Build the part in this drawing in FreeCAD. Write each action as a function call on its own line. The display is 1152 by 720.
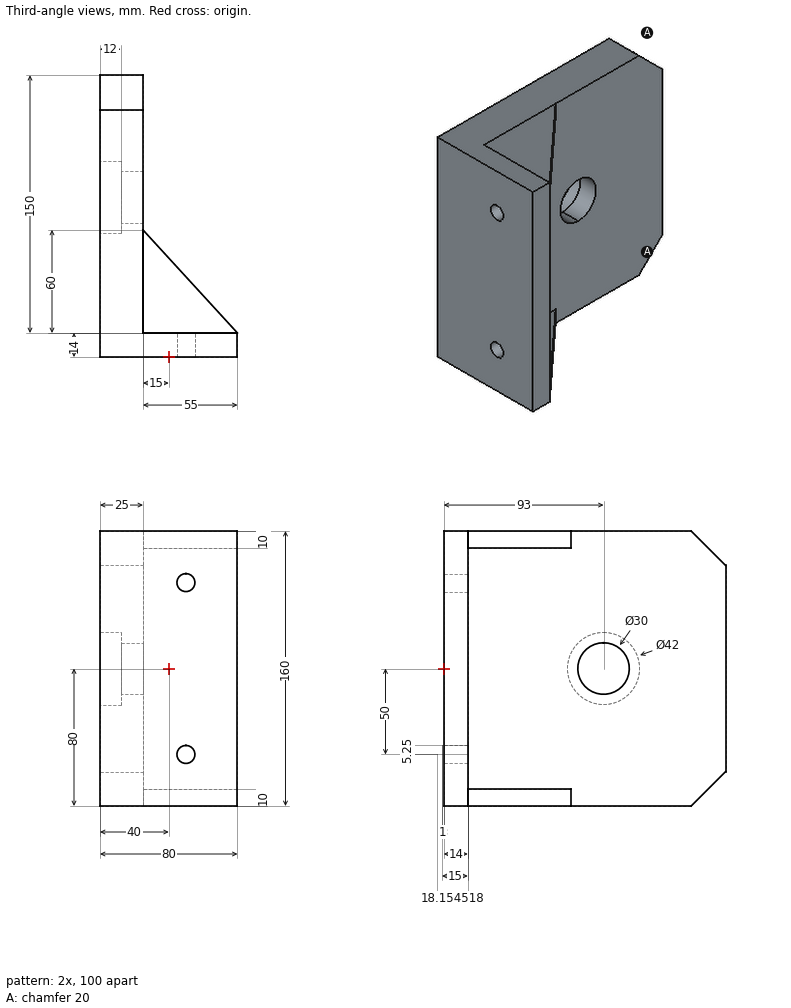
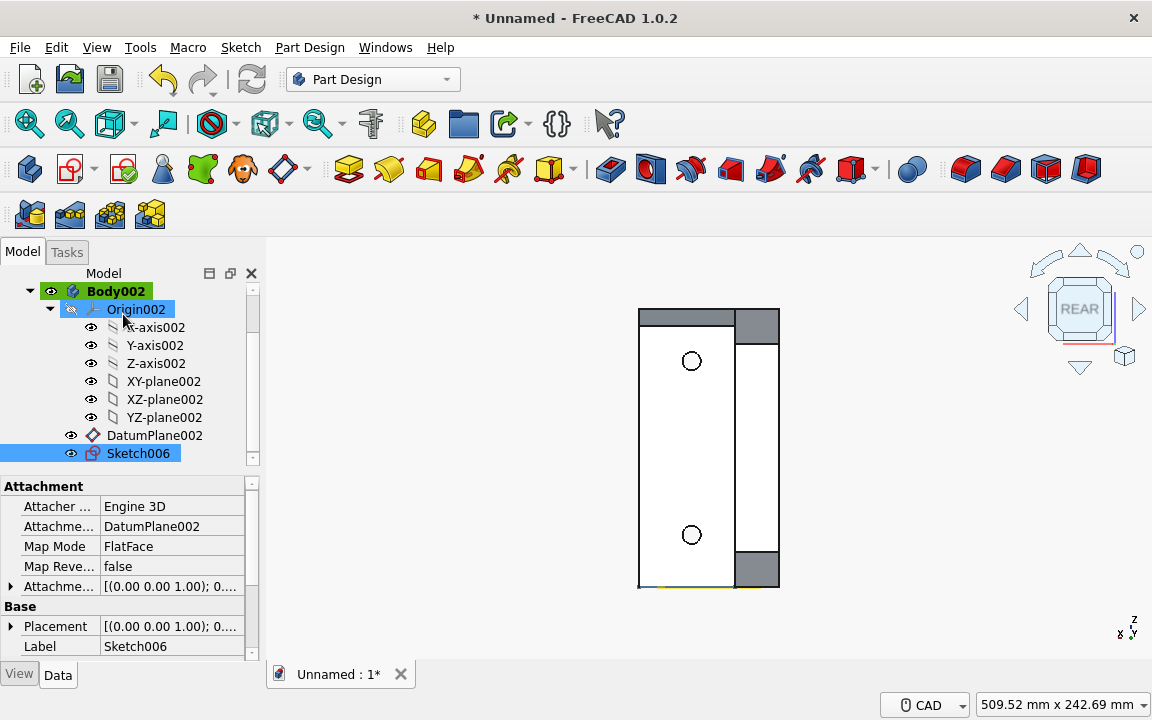
click(350, 170)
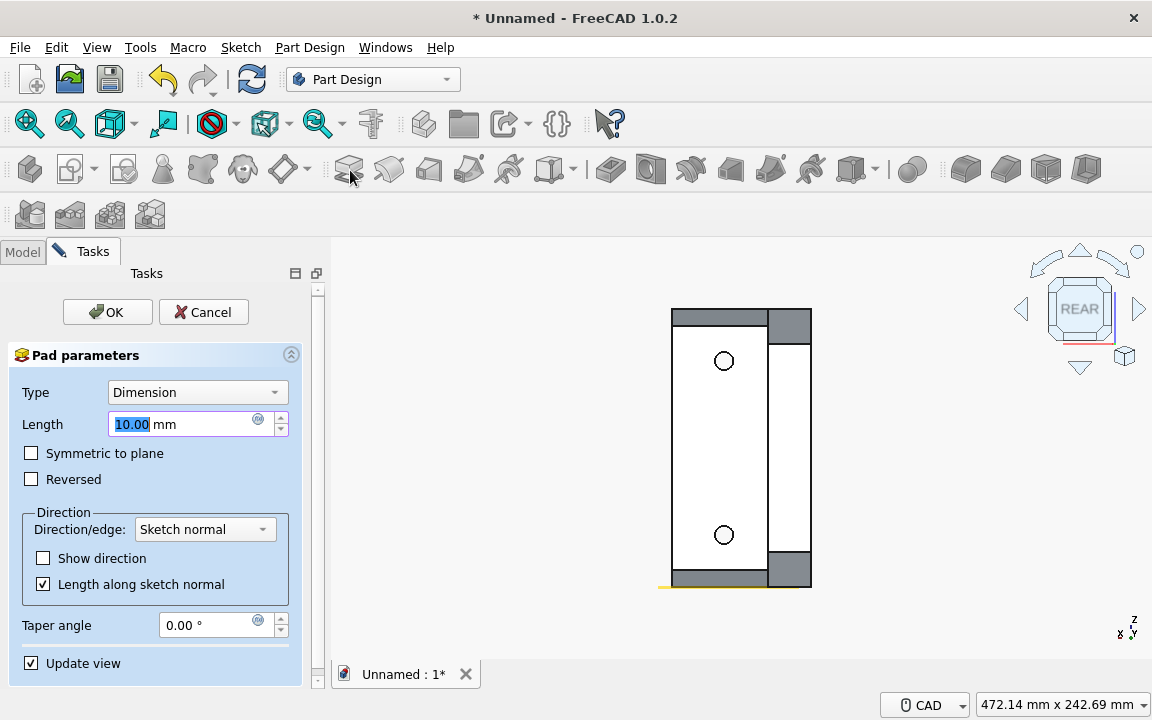
text(10)
key(Tab)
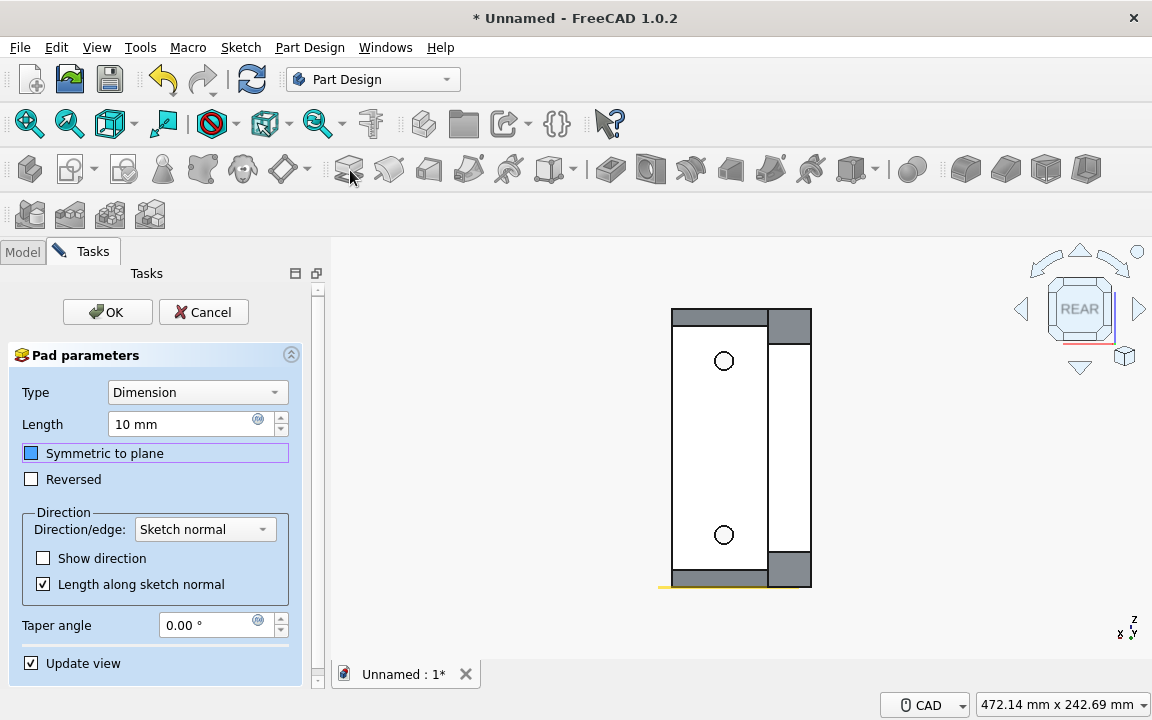
click(108, 312)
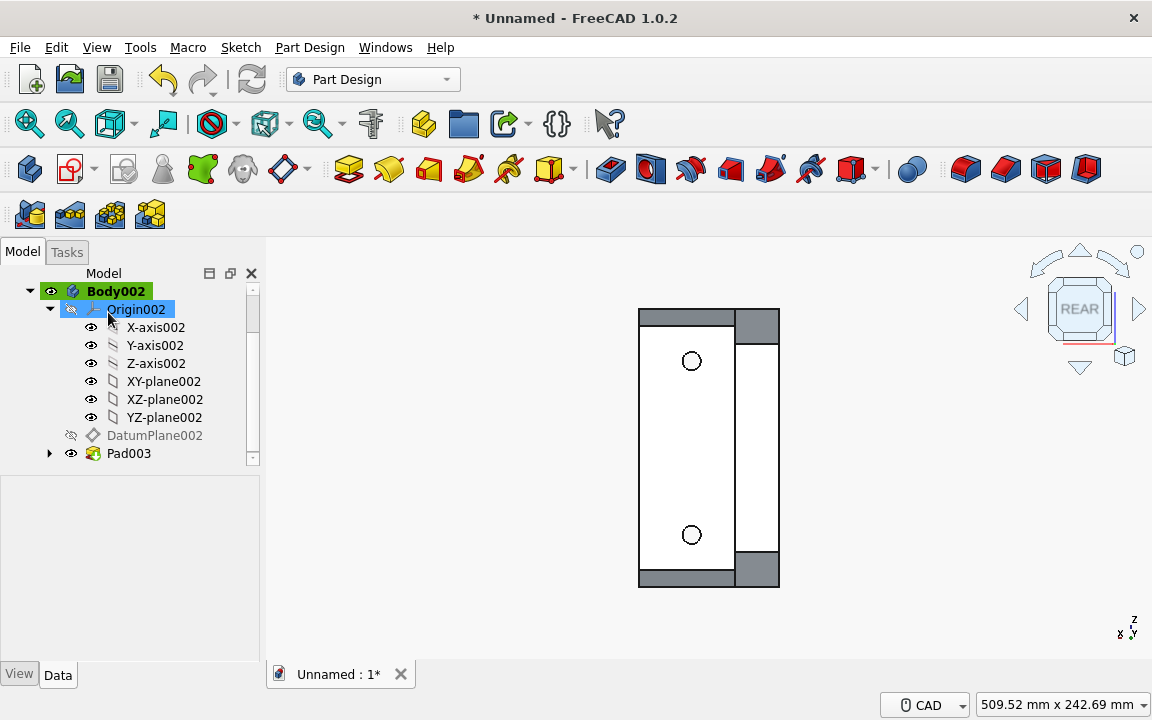
key(0)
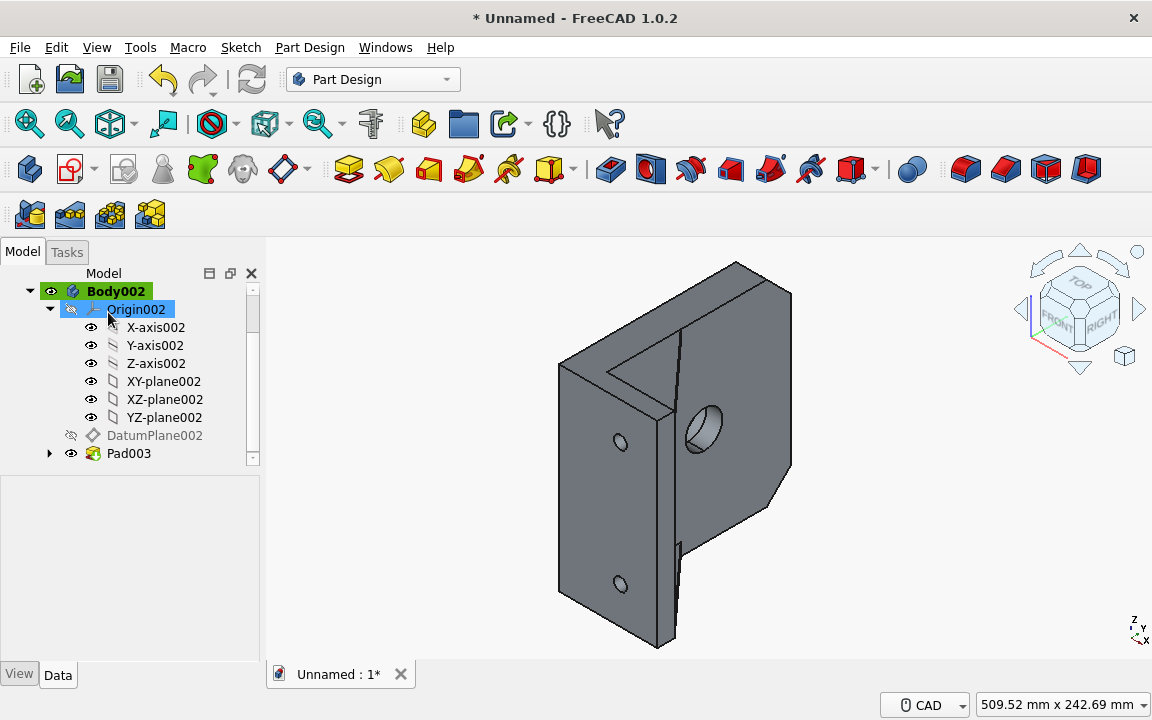
key(v)
key(f)